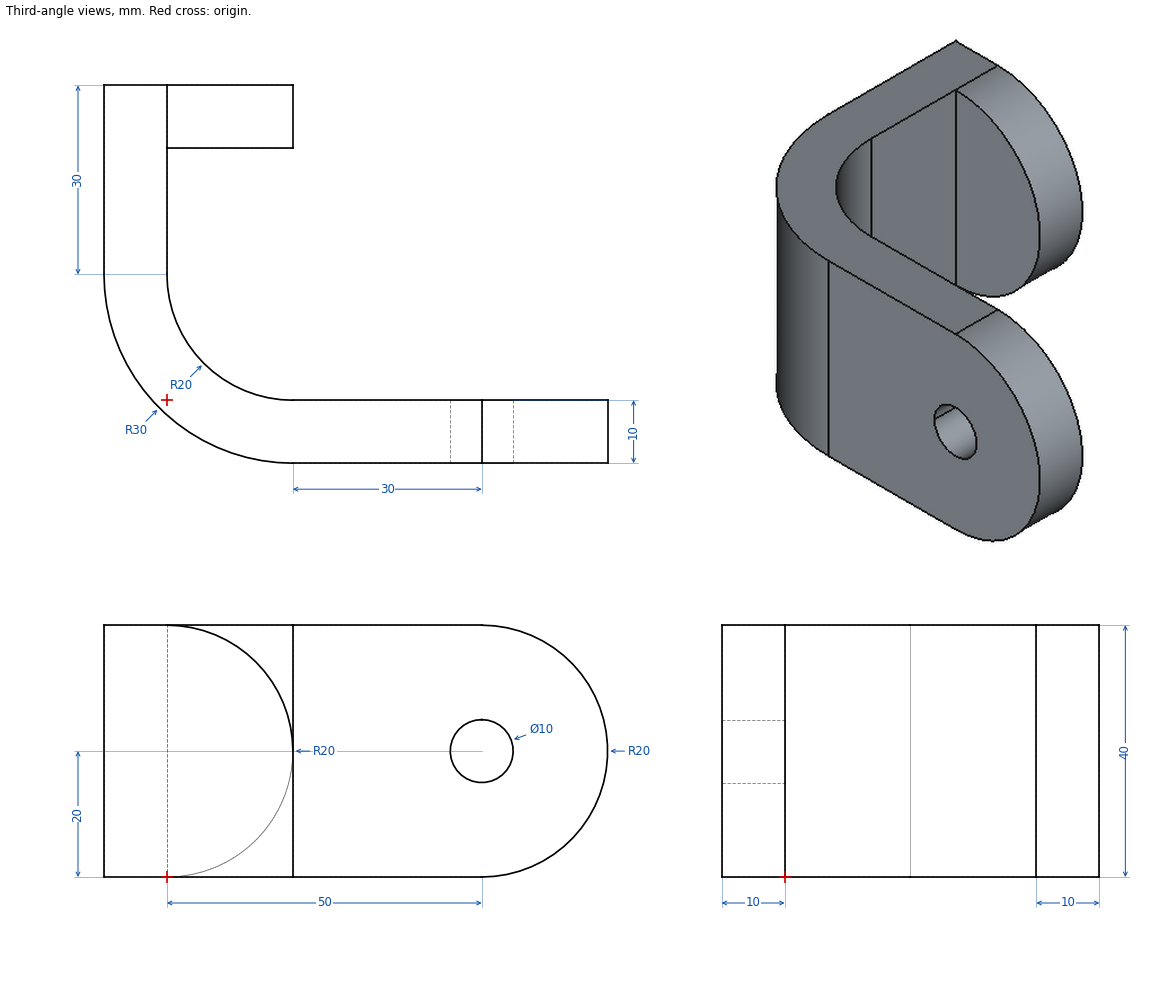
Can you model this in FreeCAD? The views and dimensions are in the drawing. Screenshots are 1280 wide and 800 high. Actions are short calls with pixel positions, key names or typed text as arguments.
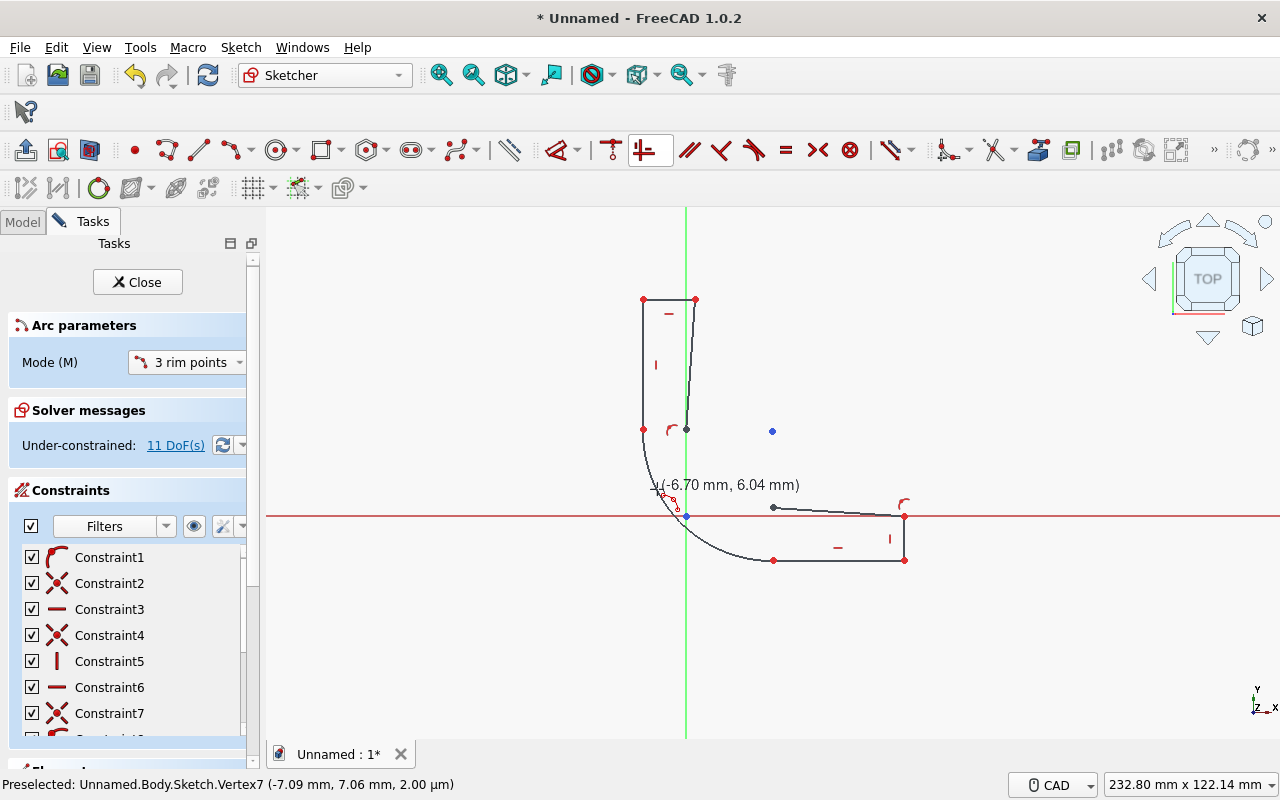
click(773, 508)
click(686, 430)
click(712, 491)
key(Escape)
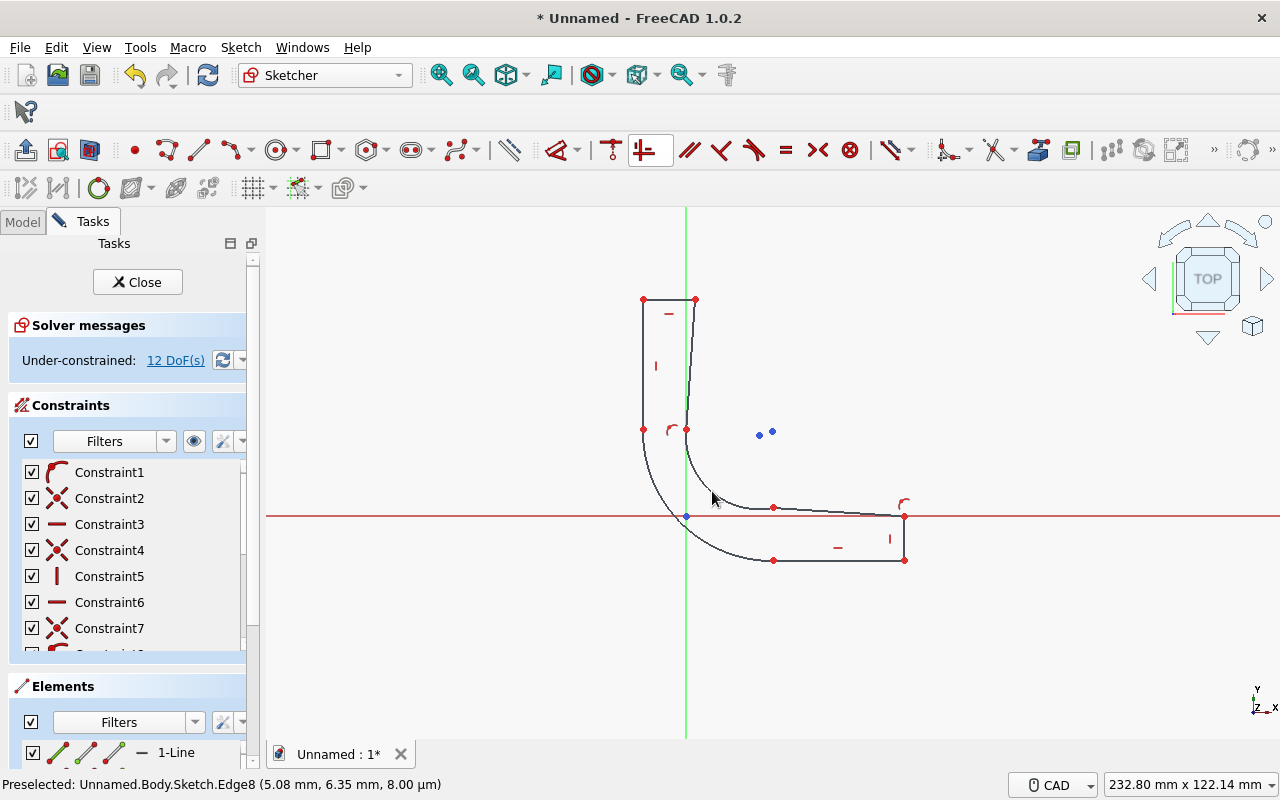
click(689, 391)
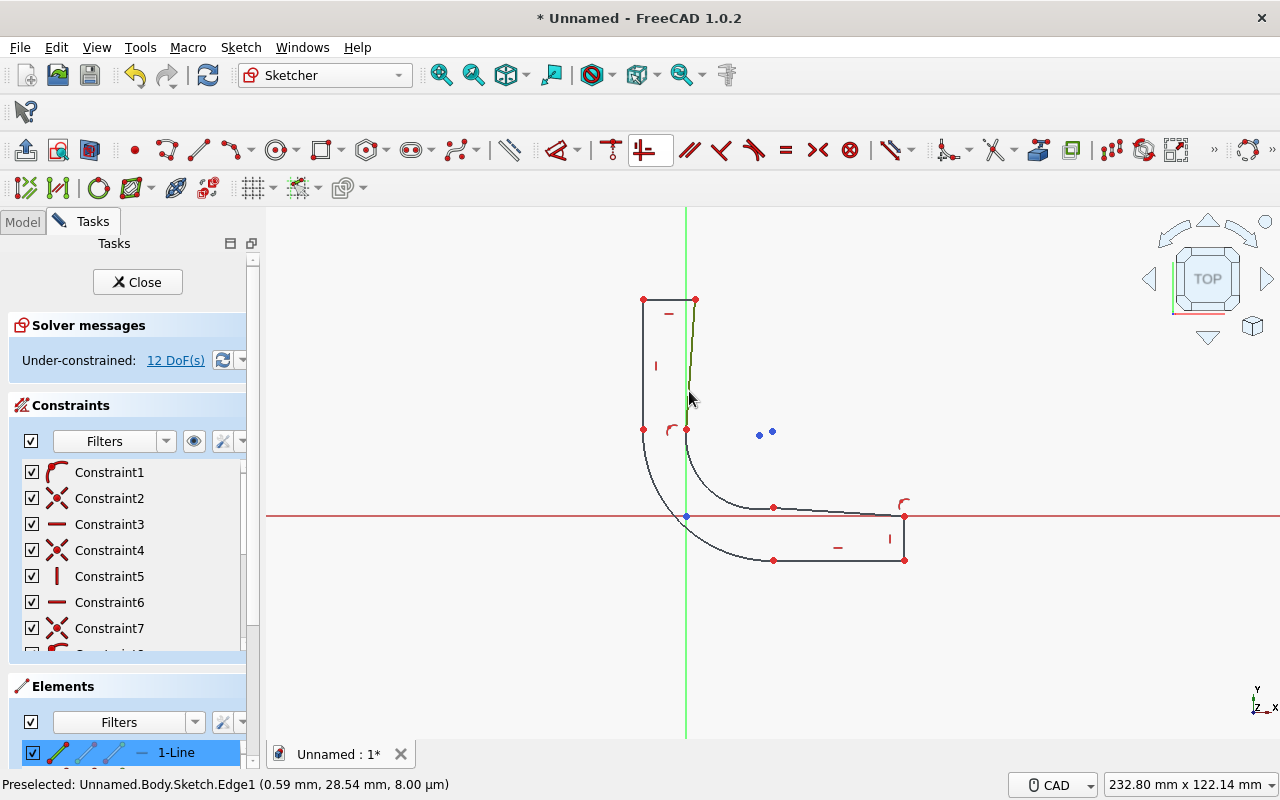
click(733, 504)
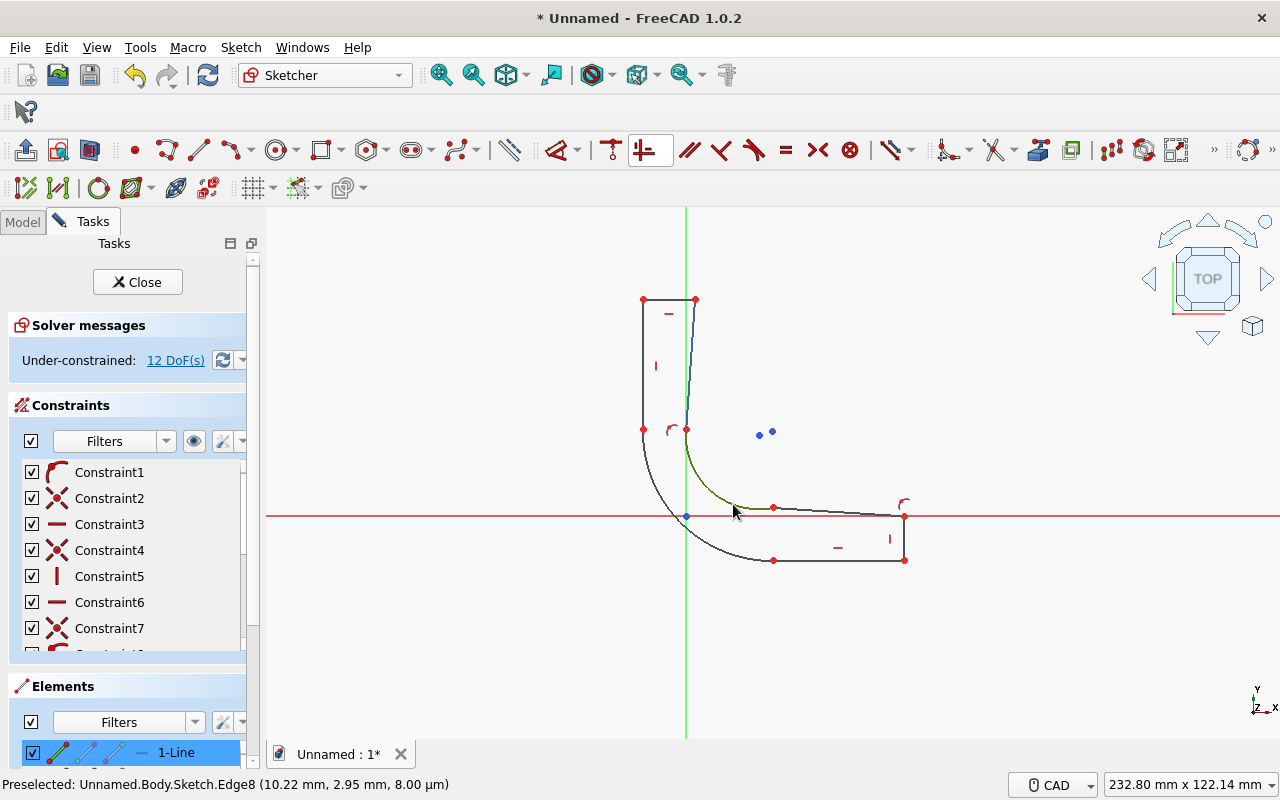
key(t)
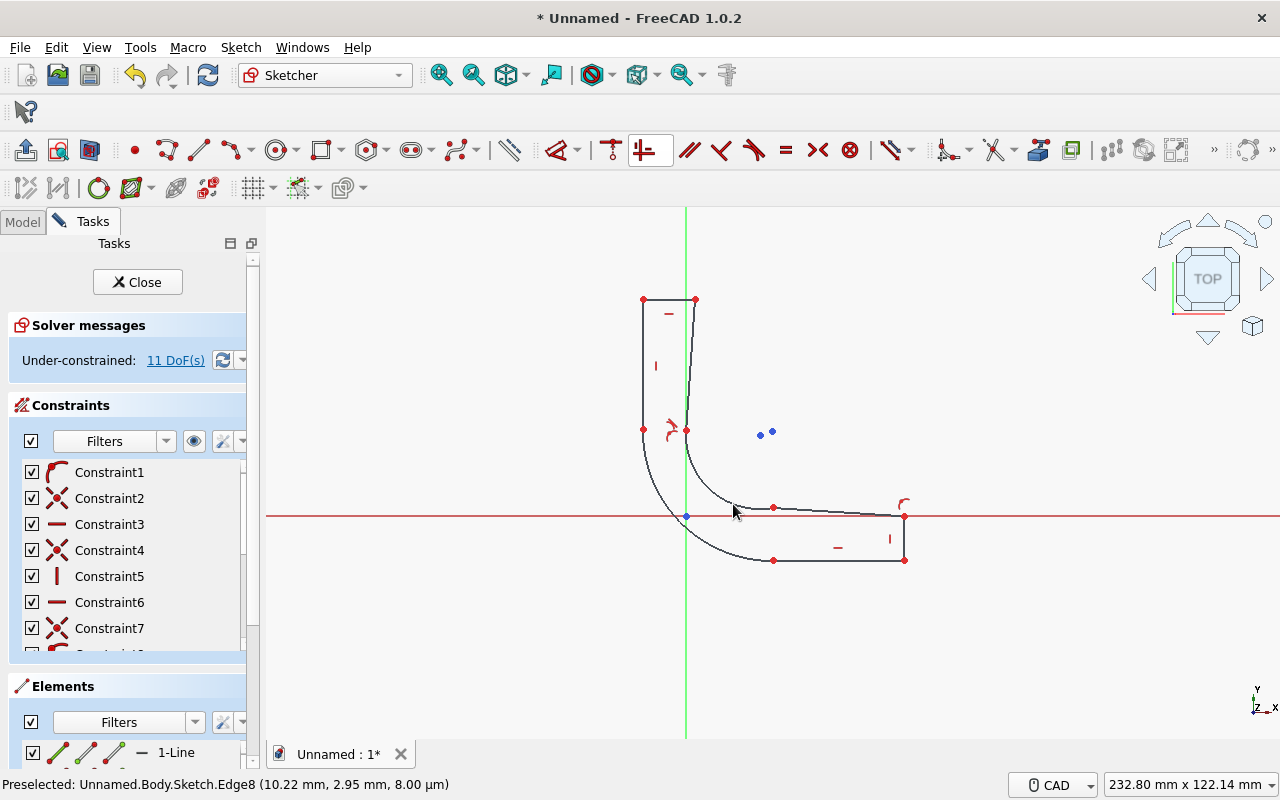
click(643, 339)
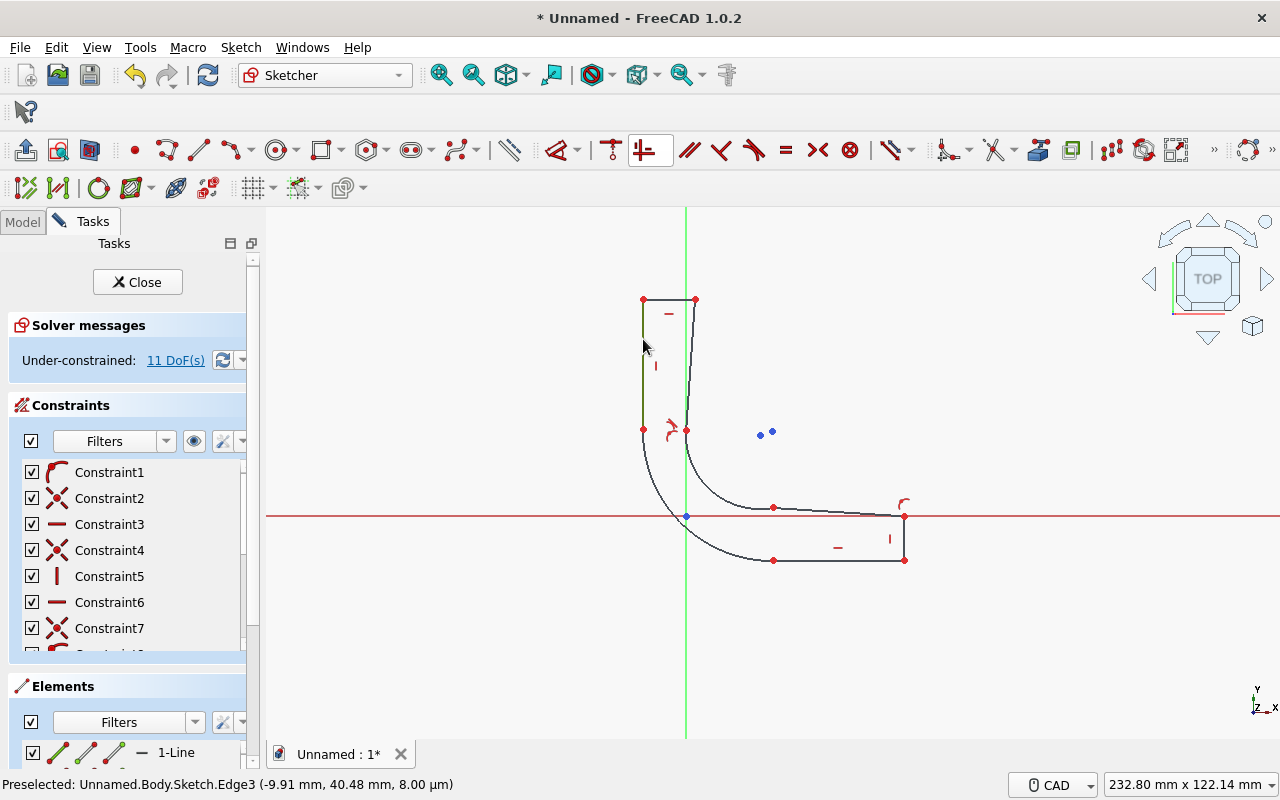
click(657, 489)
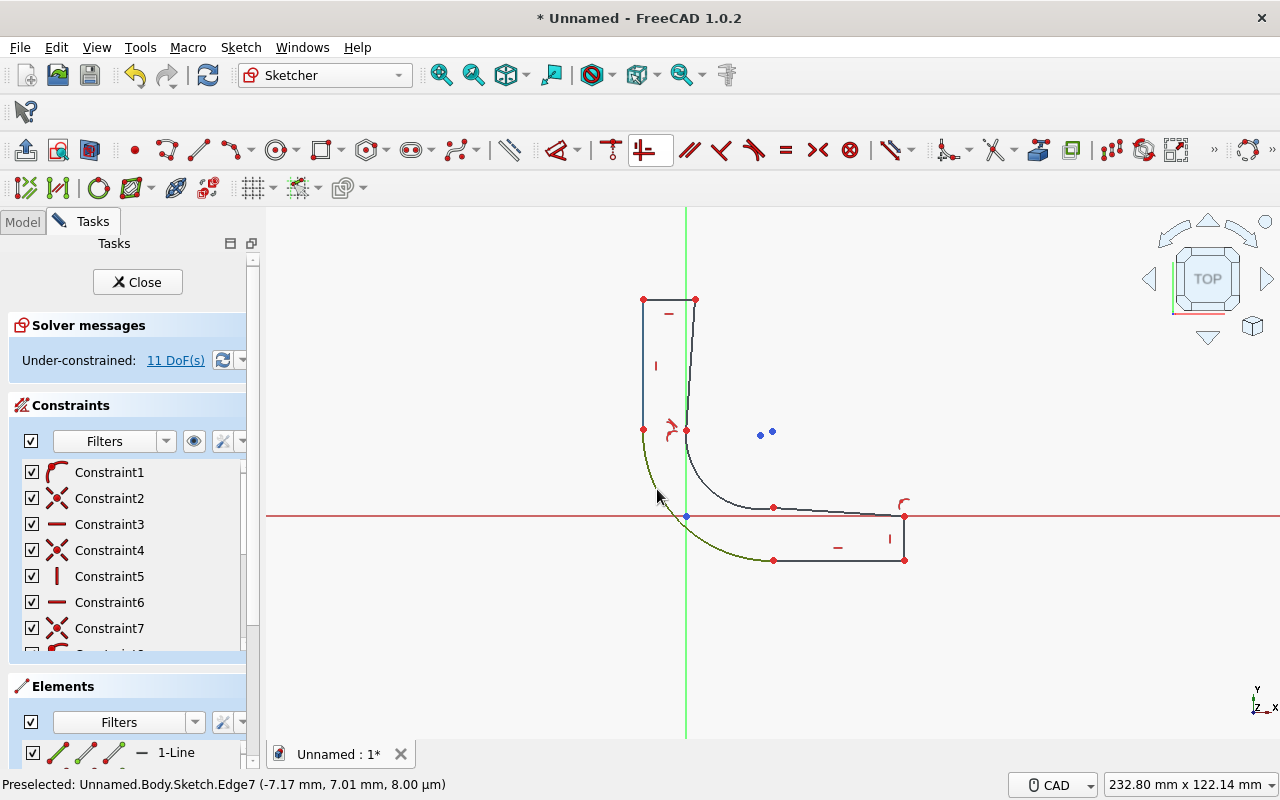
key(t)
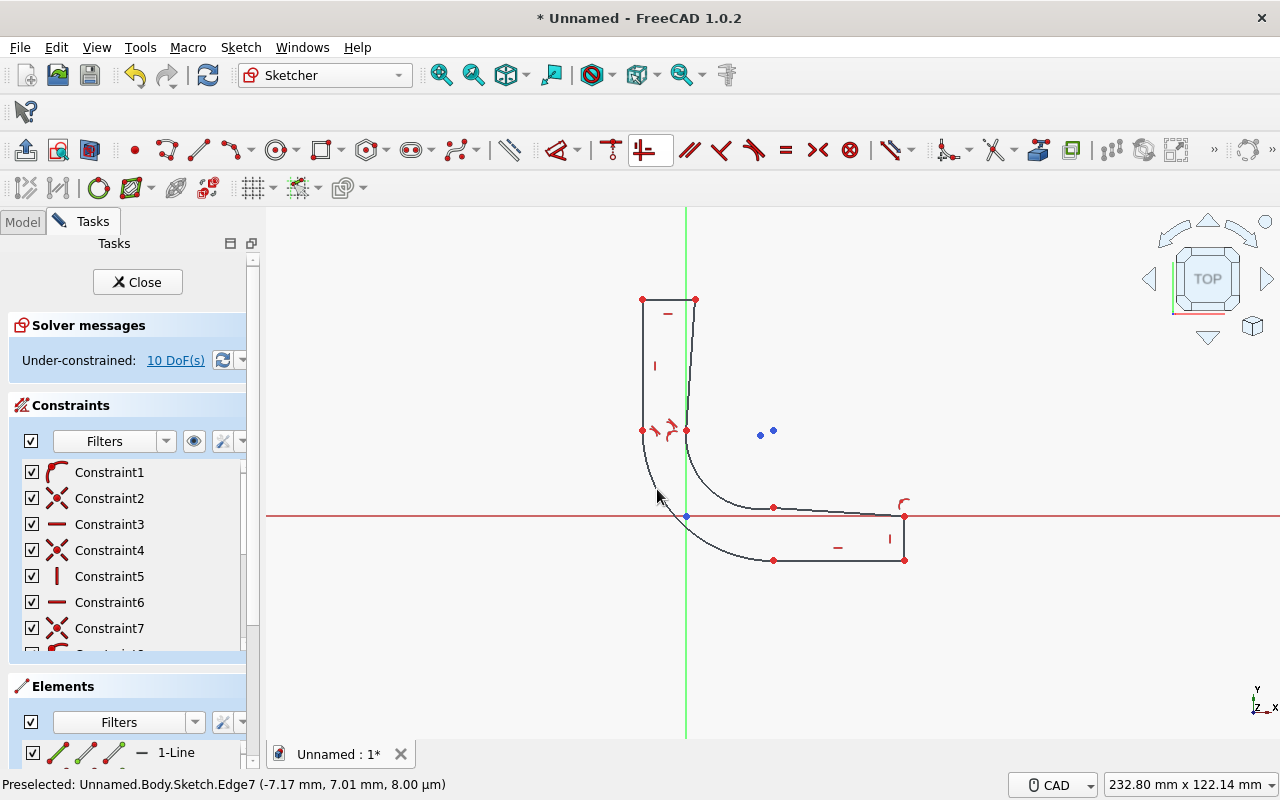
click(812, 561)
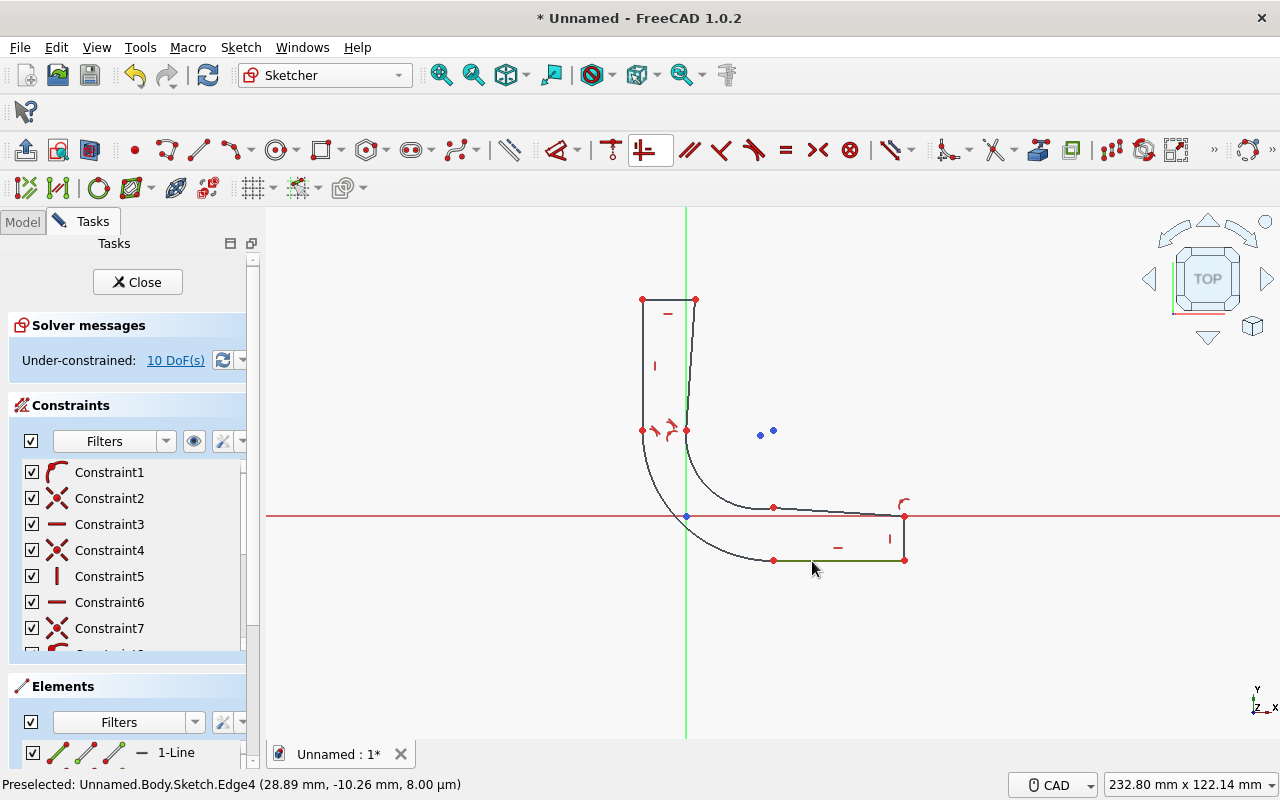
click(657, 489)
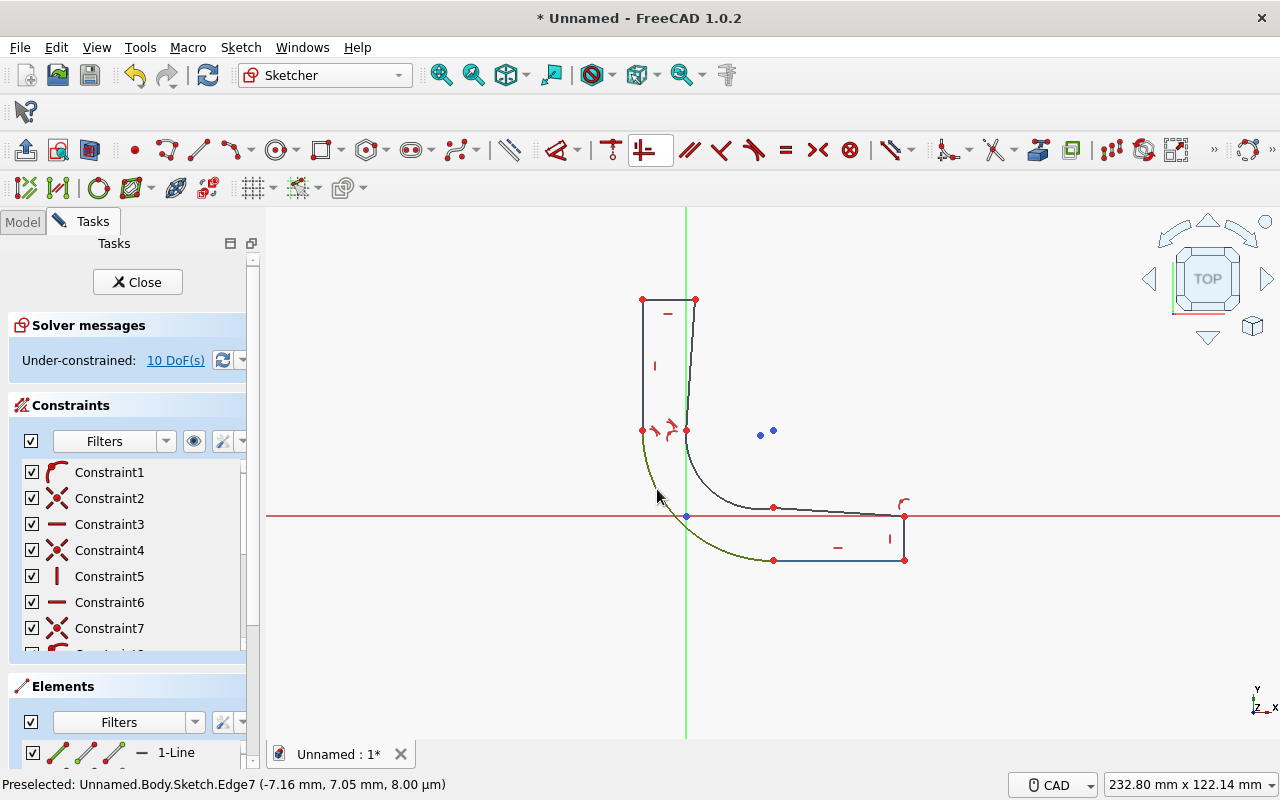
click(754, 150)